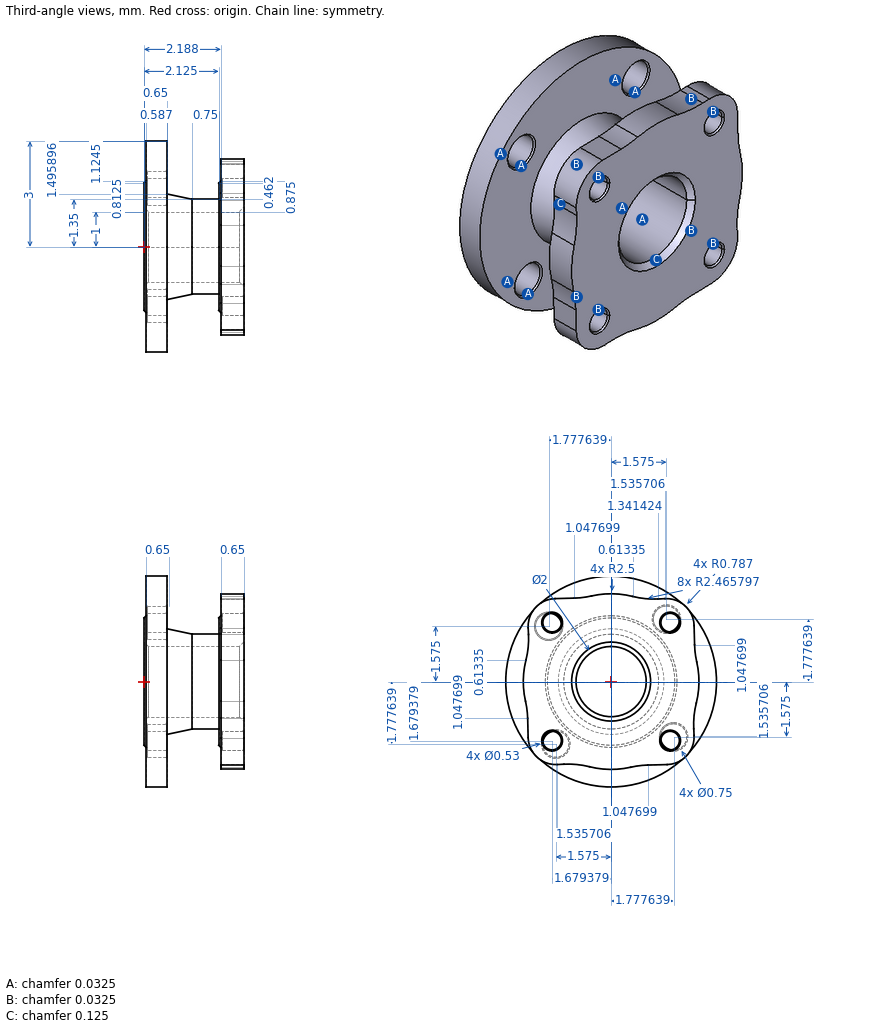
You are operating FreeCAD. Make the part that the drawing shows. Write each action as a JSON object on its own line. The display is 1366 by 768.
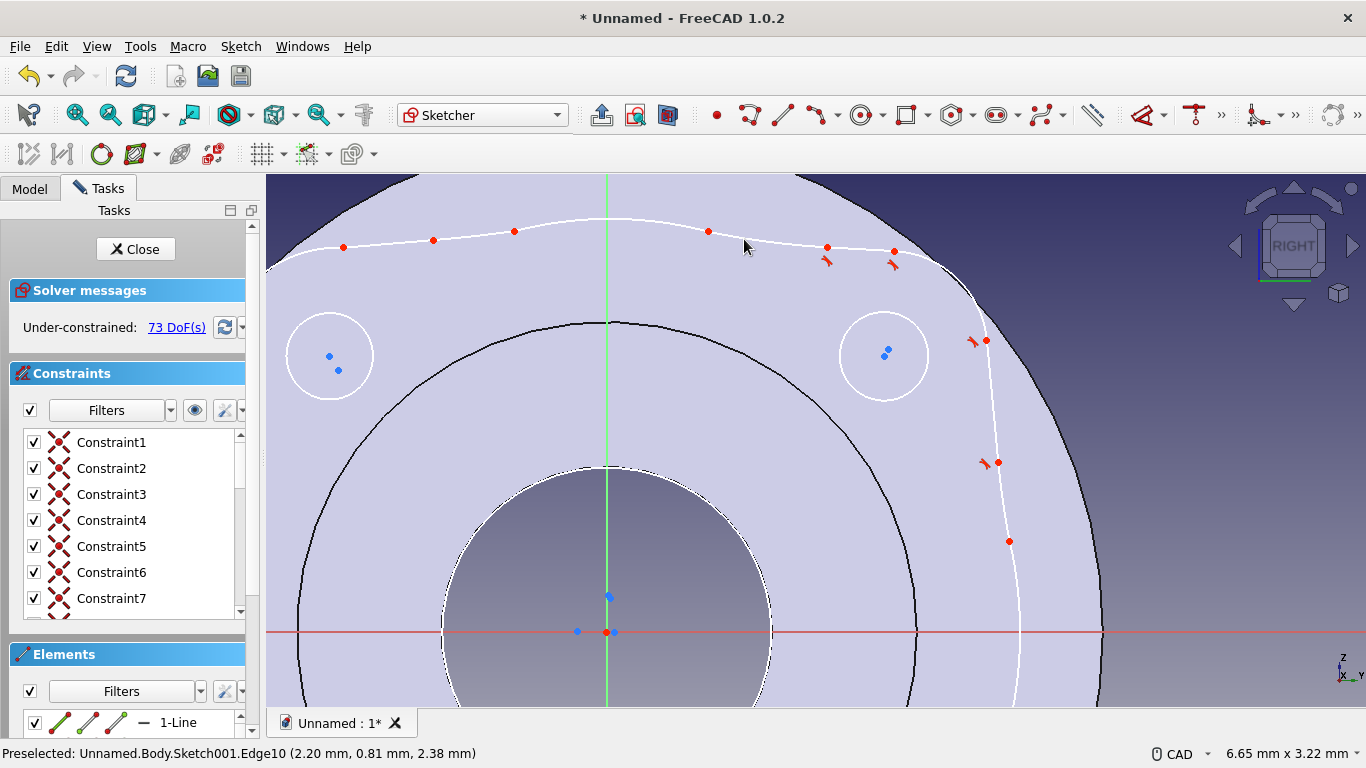
{"action": "left_click", "coordinate": [406, 242]}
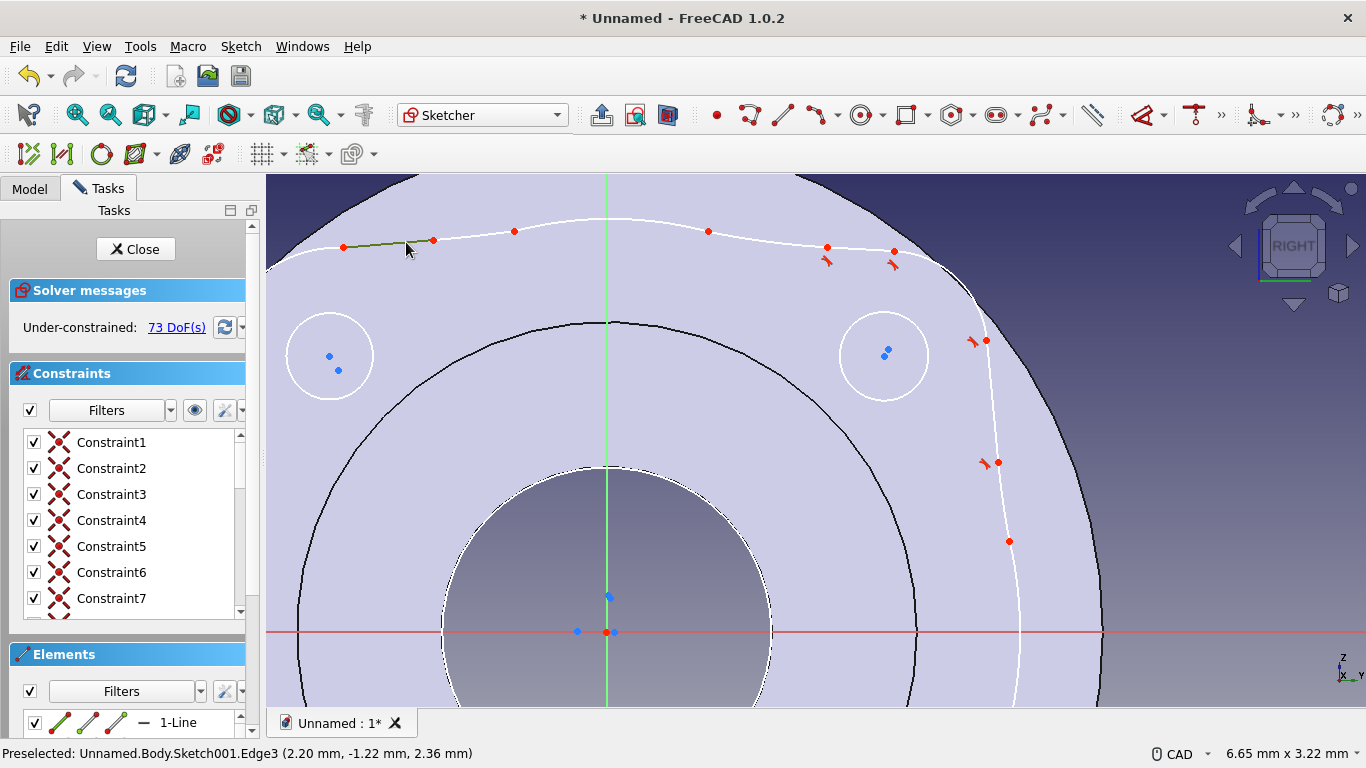
{"action": "left_click", "coordinate": [458, 238]}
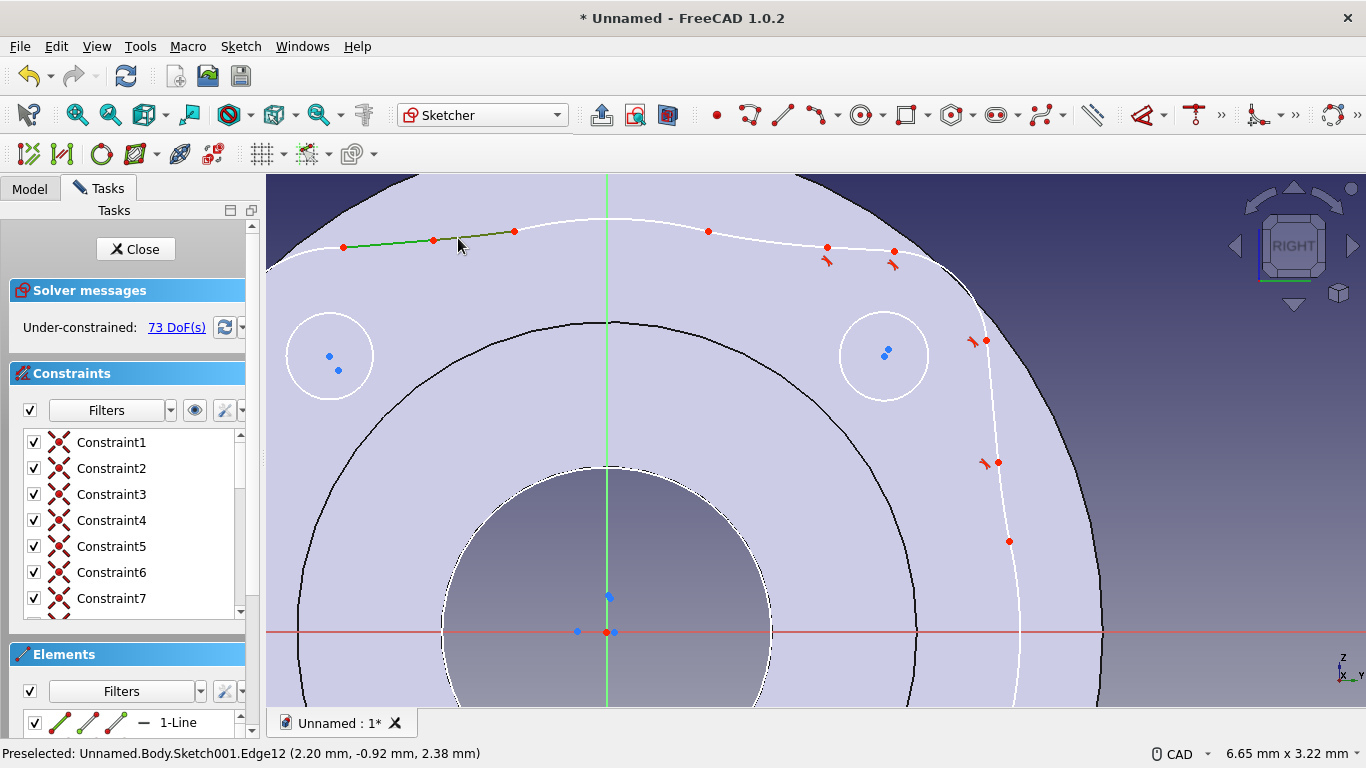
{"action": "key", "text": "t"}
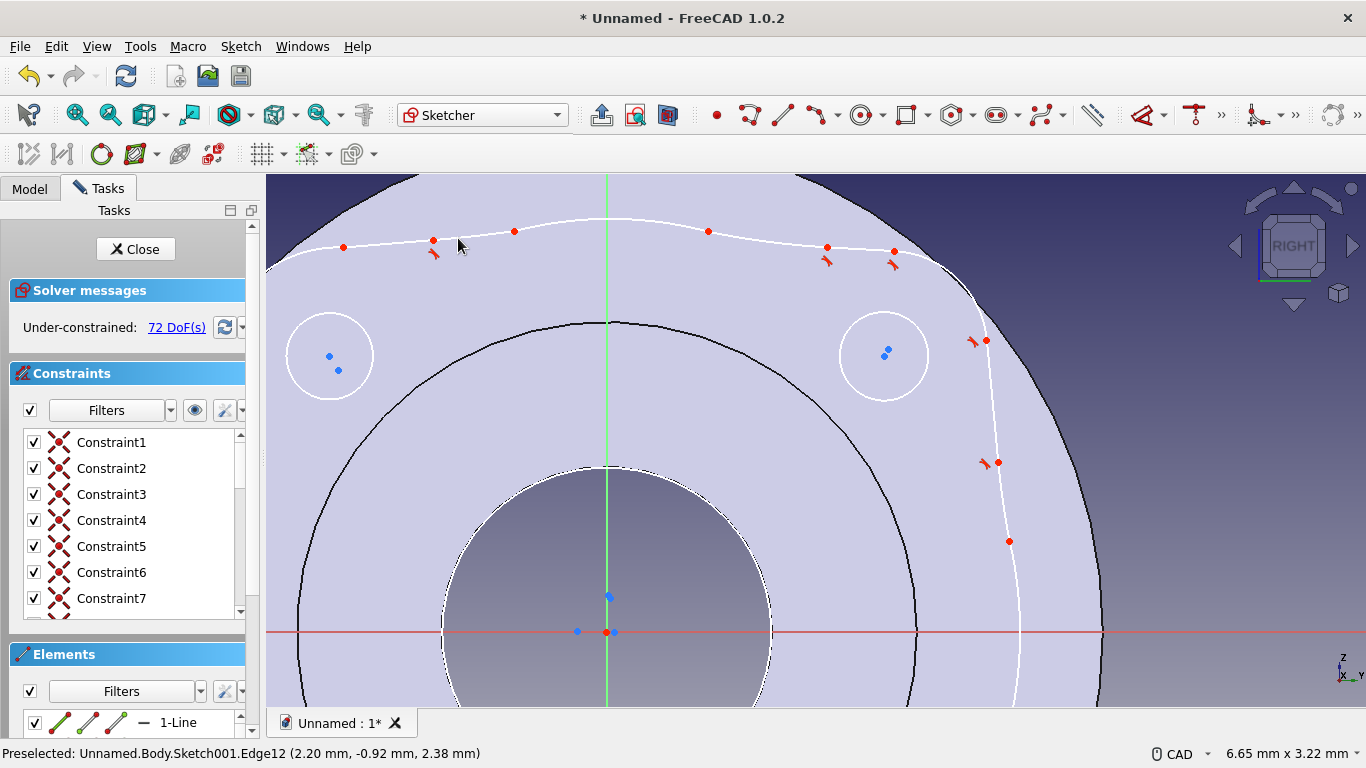
{"action": "left_click", "coordinate": [406, 242]}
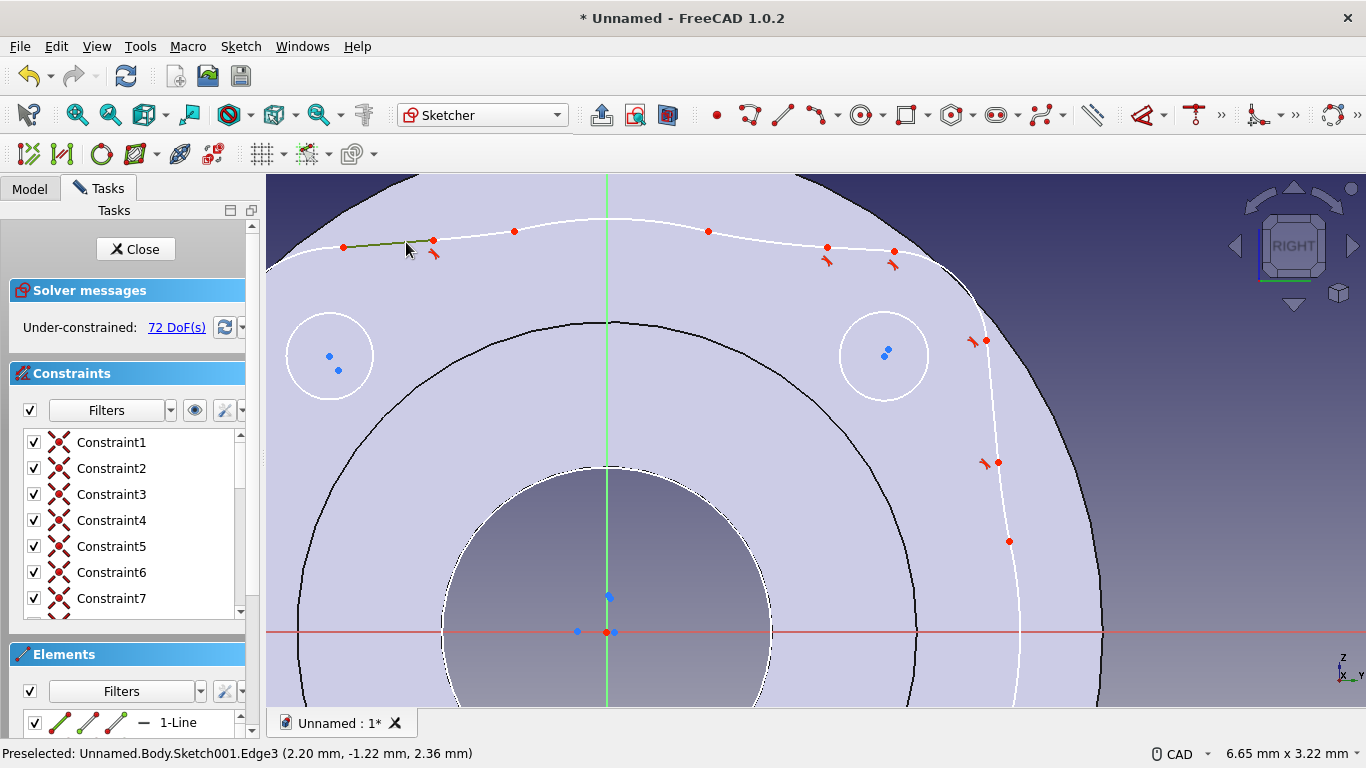
{"action": "left_click", "coordinate": [303, 253]}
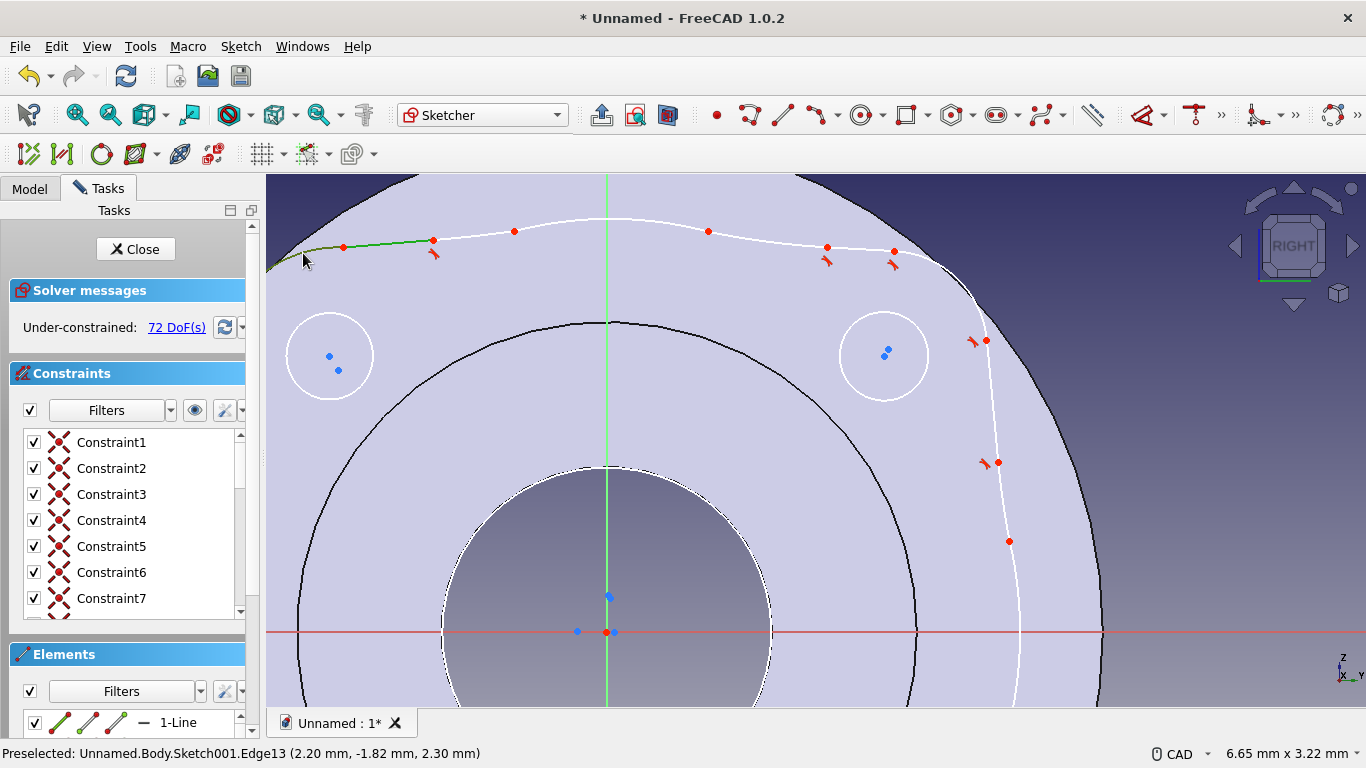
{"action": "key", "text": "t"}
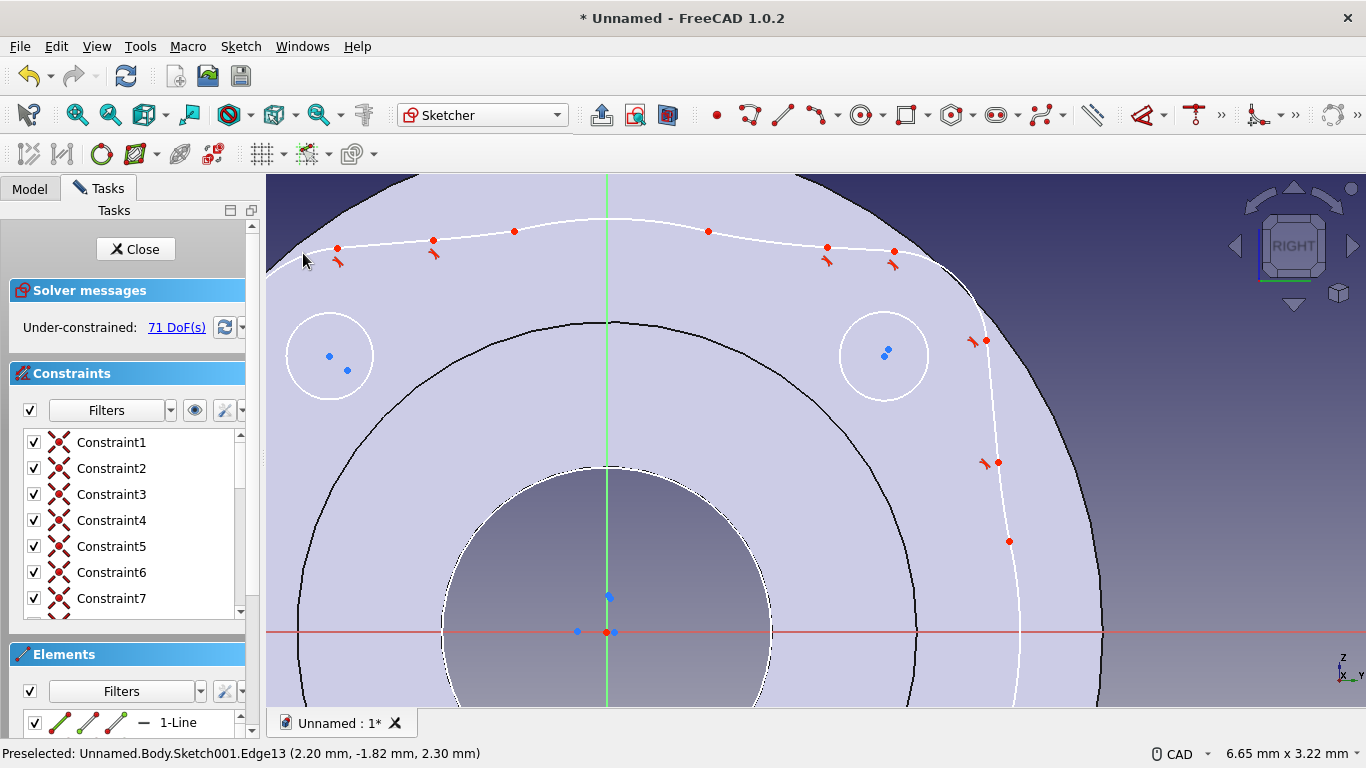
{"action": "scroll", "coordinate": [862, 284], "scroll_direction": "down", "scroll_amount": 4}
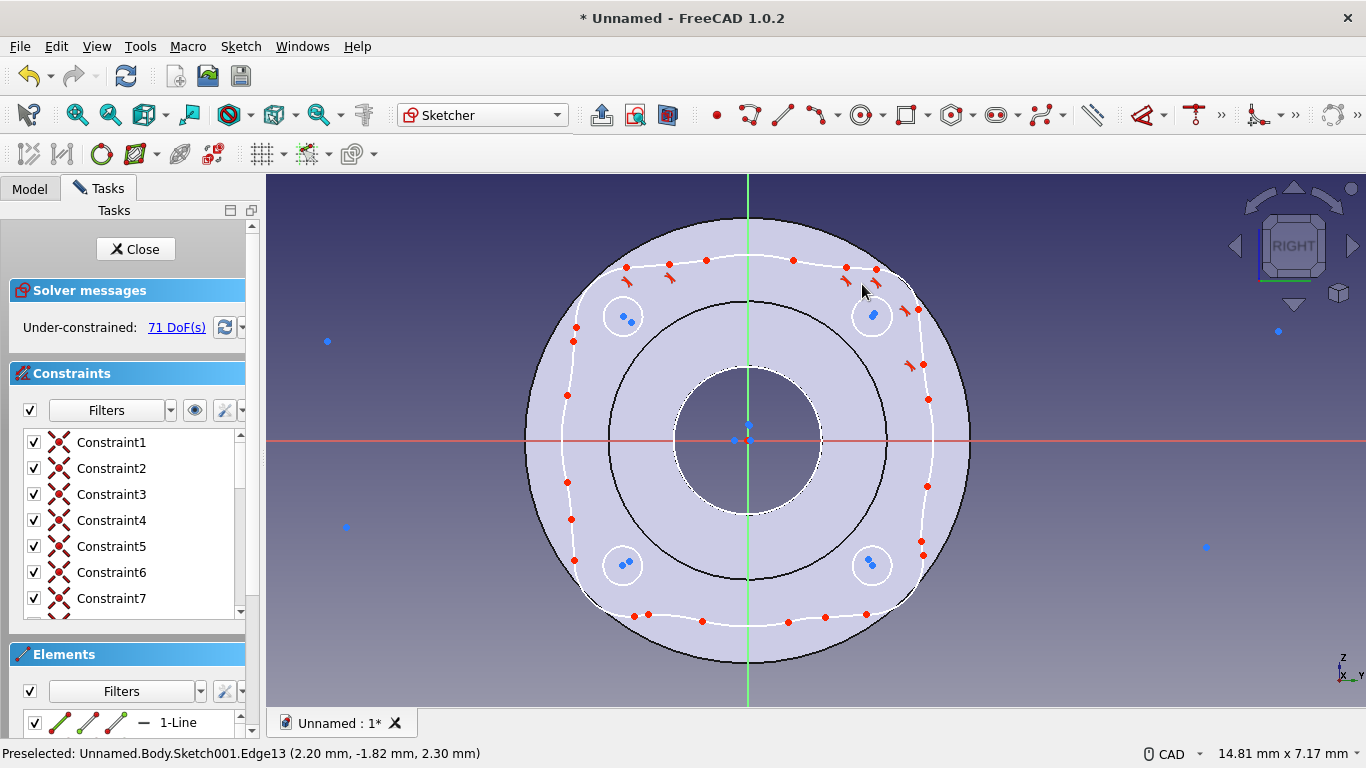
{"action": "scroll", "coordinate": [575, 332], "scroll_direction": "up", "scroll_amount": 6}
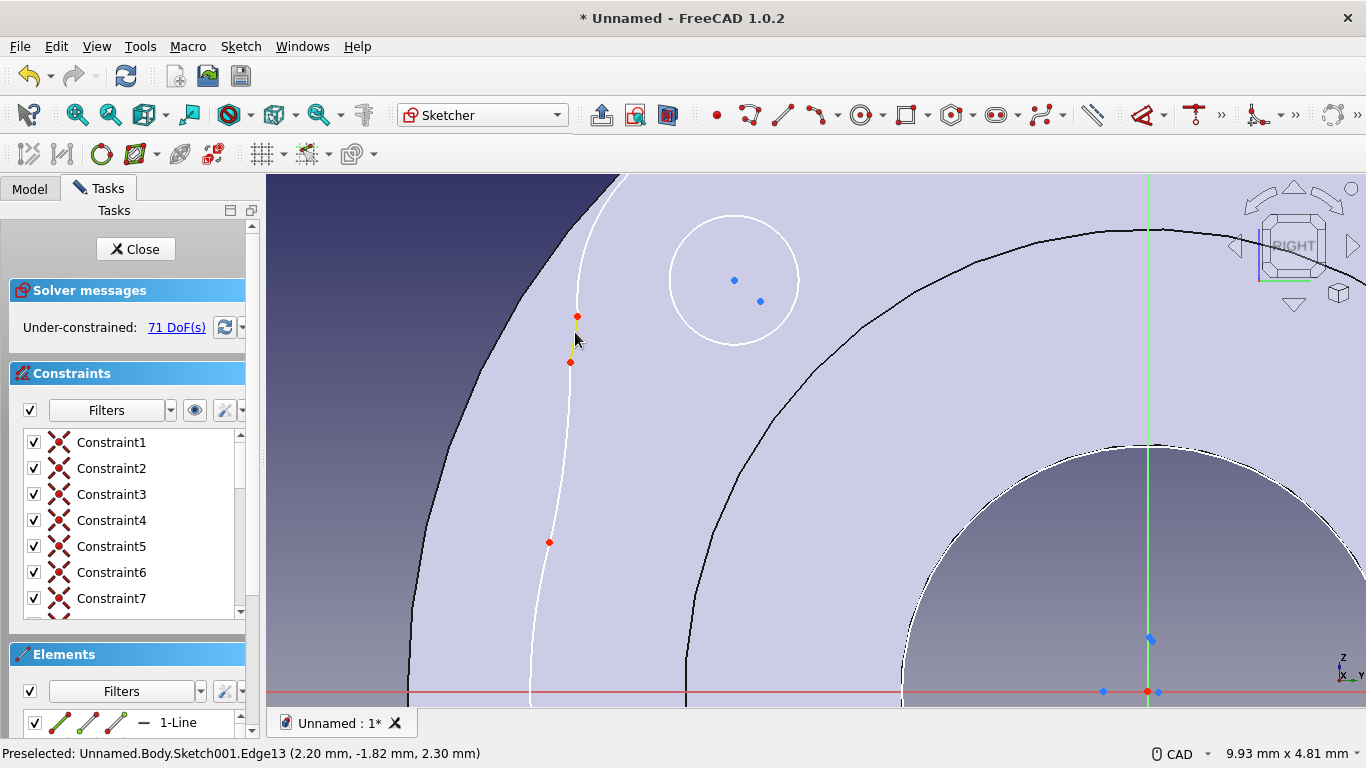
{"action": "left_click", "coordinate": [576, 331]}